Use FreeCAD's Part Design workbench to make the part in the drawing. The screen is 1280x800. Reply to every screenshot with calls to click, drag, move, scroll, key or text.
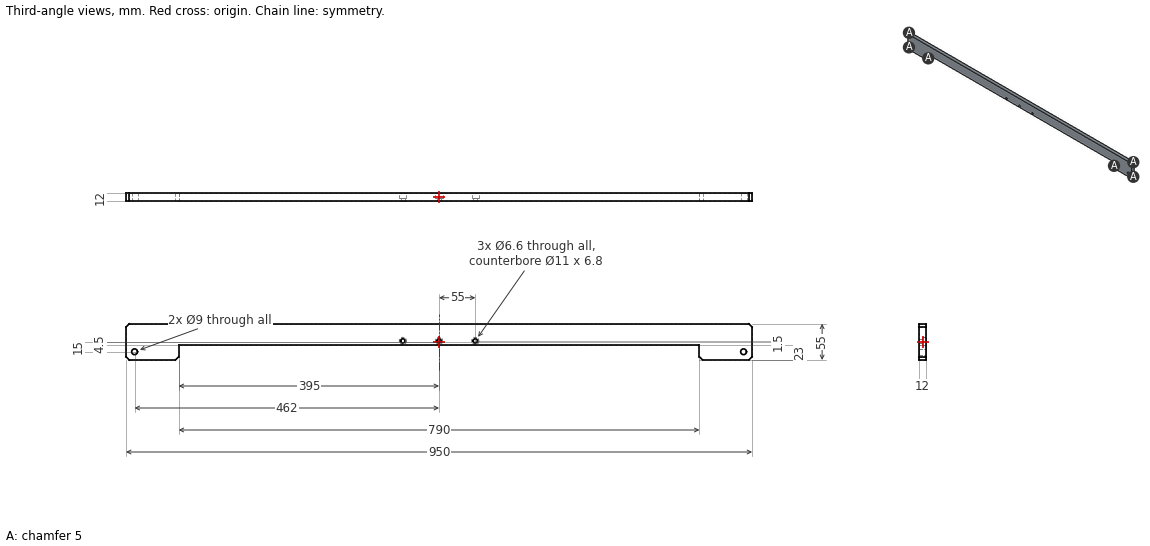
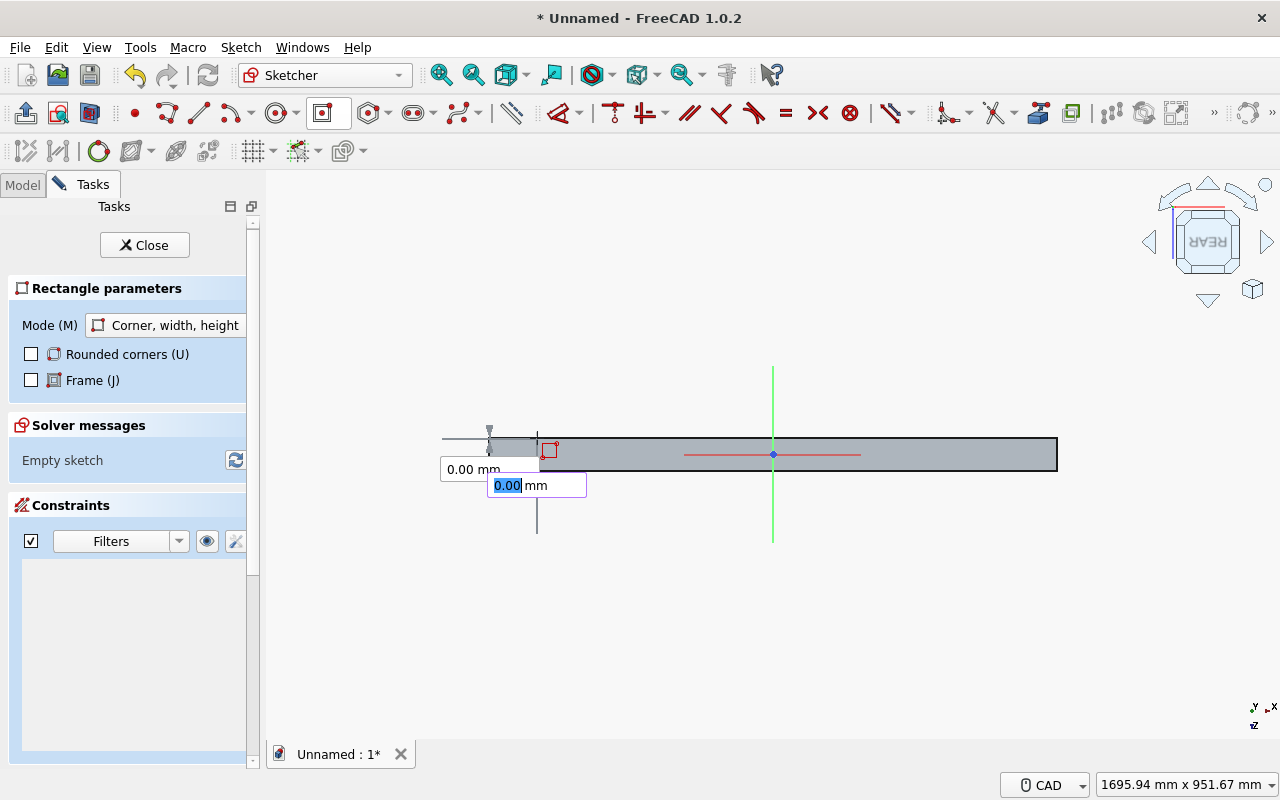
scroll(1009, 452, up, 9)
move(1006, 448)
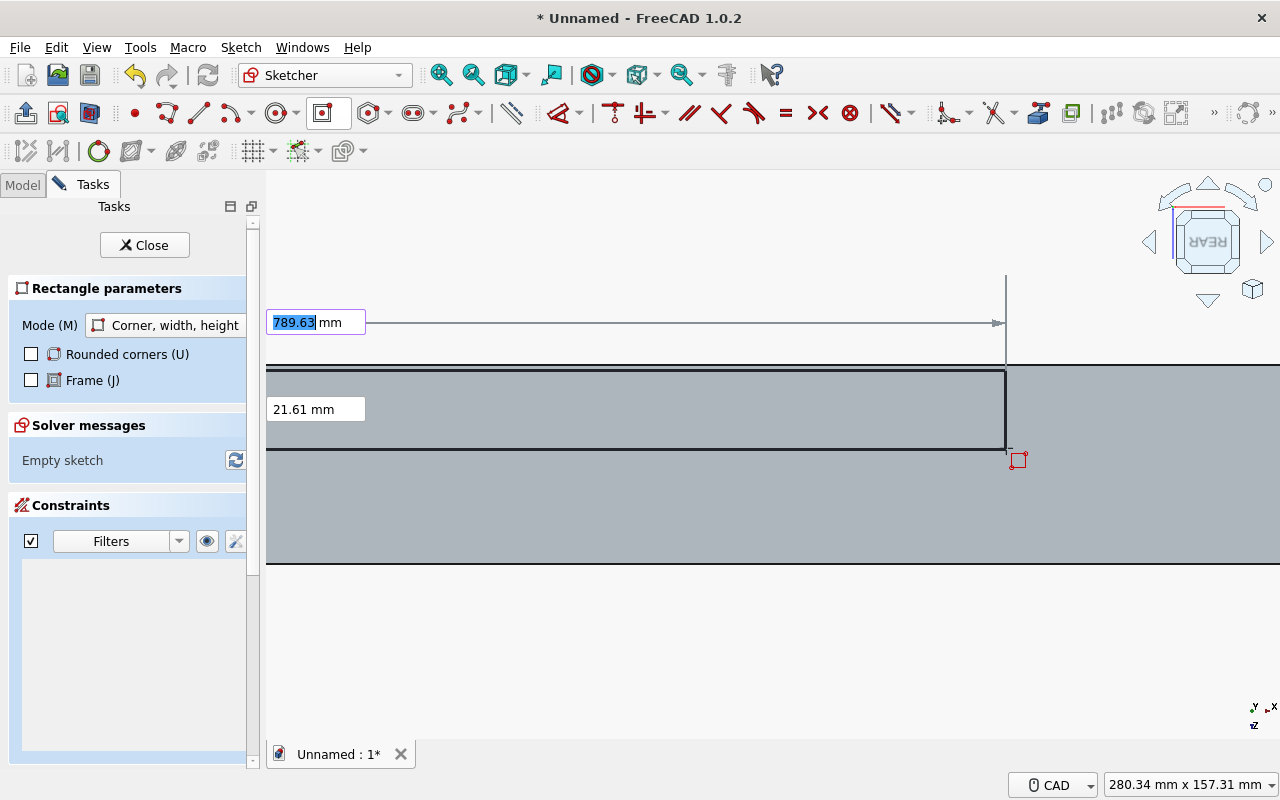
text(790)
key(Tab)
text(23)
key(Return)
key(Escape)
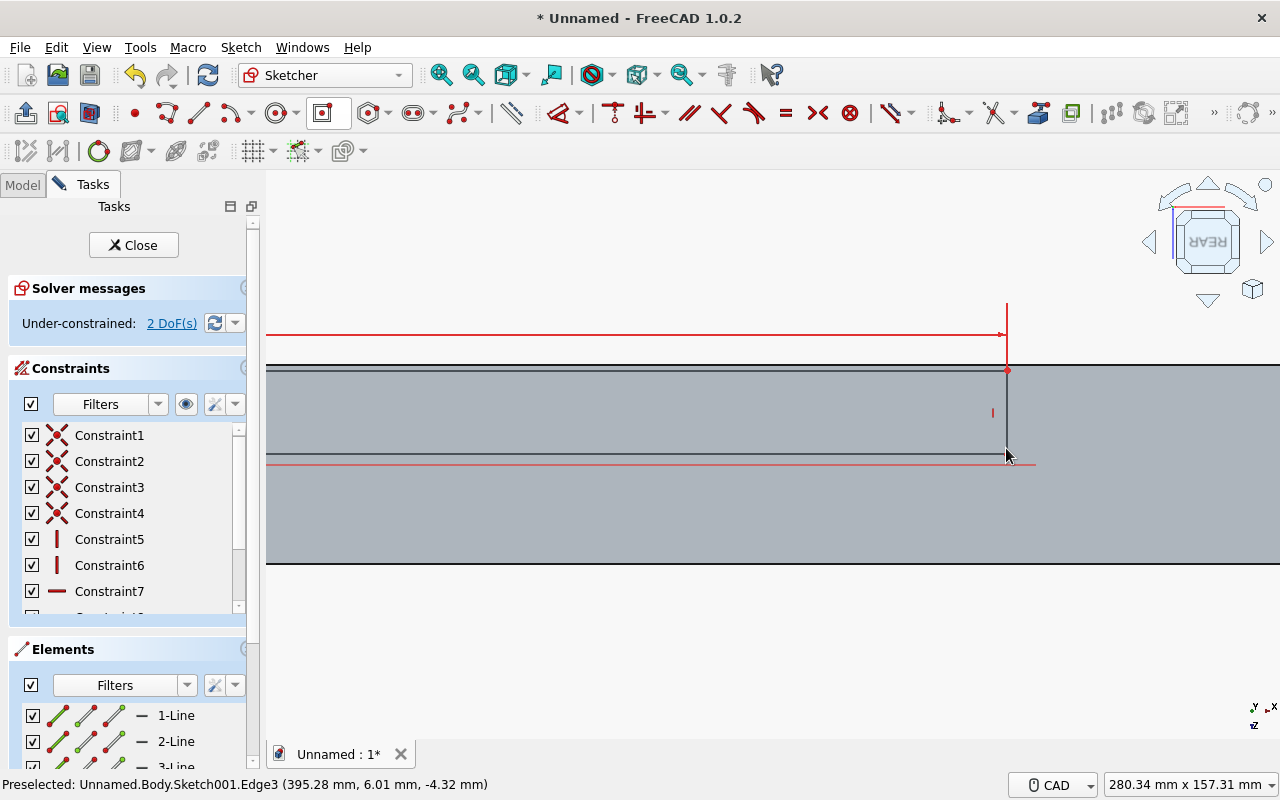
click(558, 114)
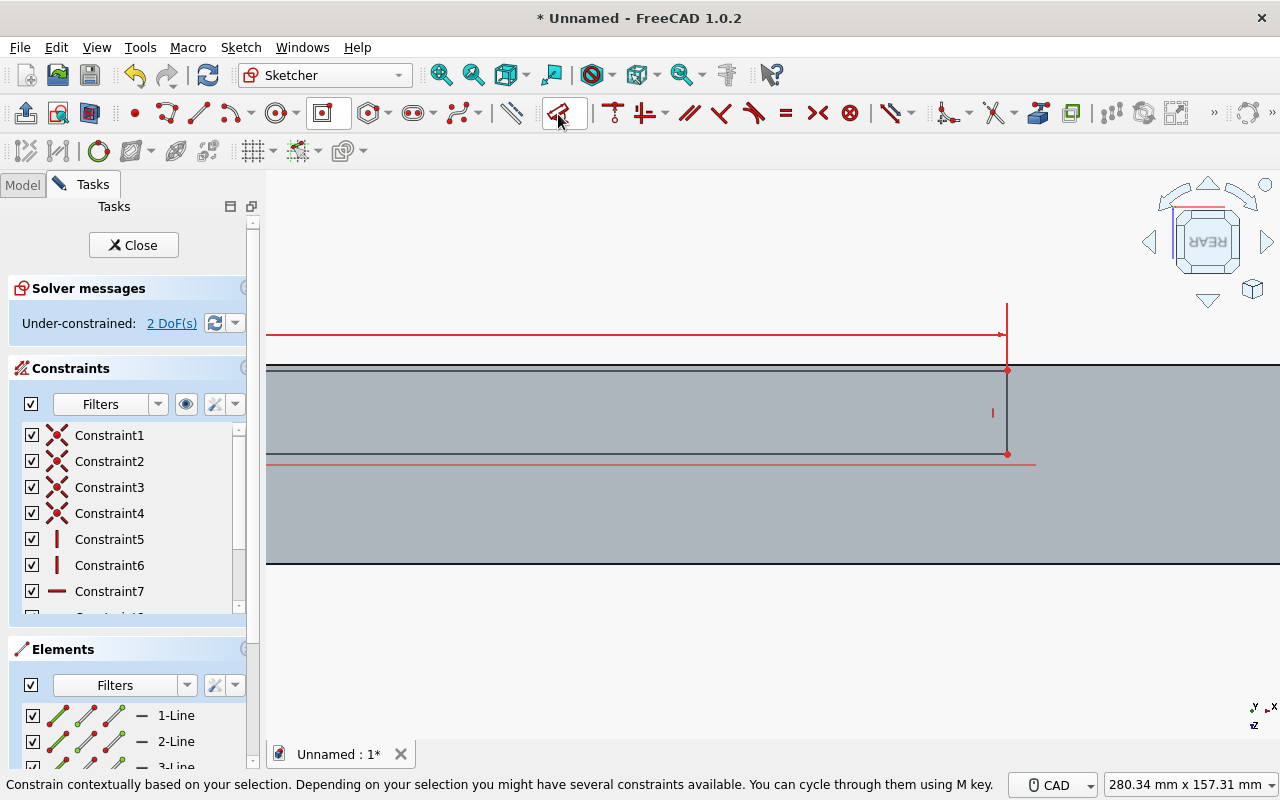
scroll(990, 465, down, 8)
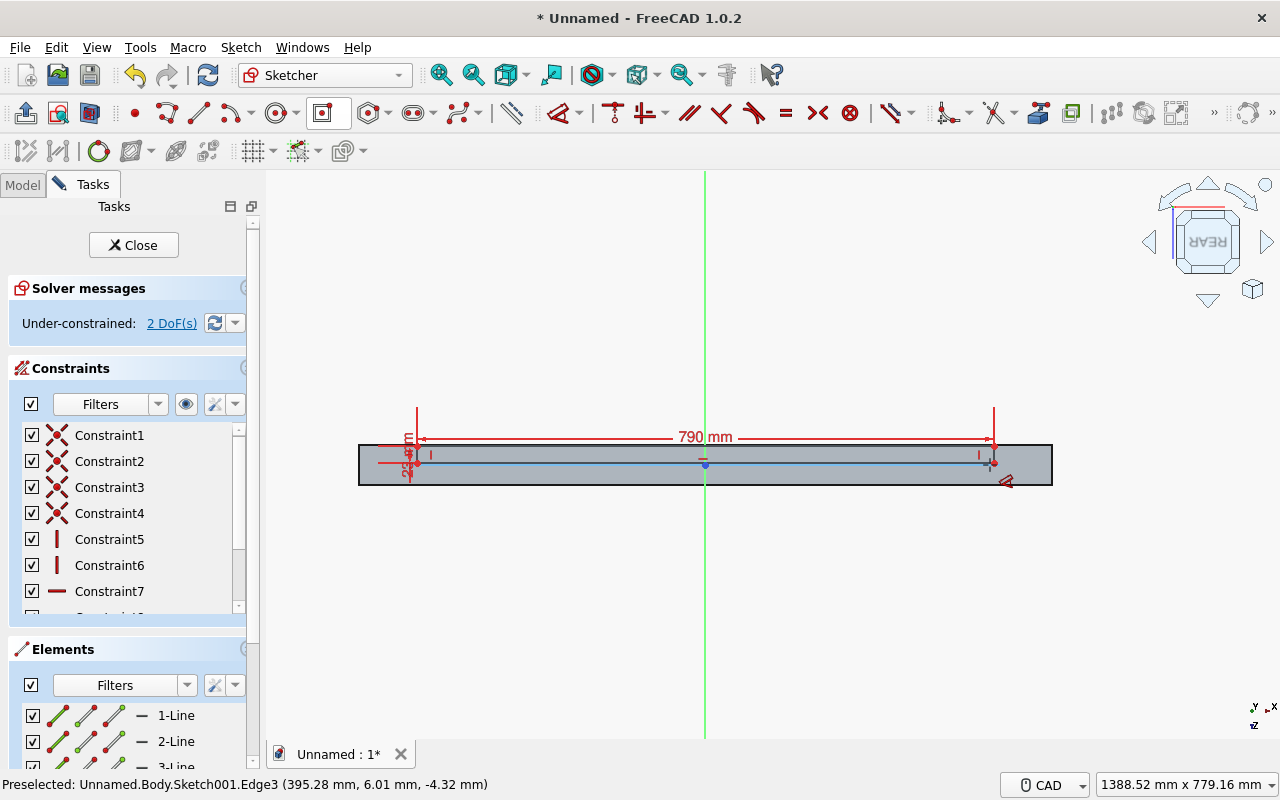
click(417, 446)
click(561, 499)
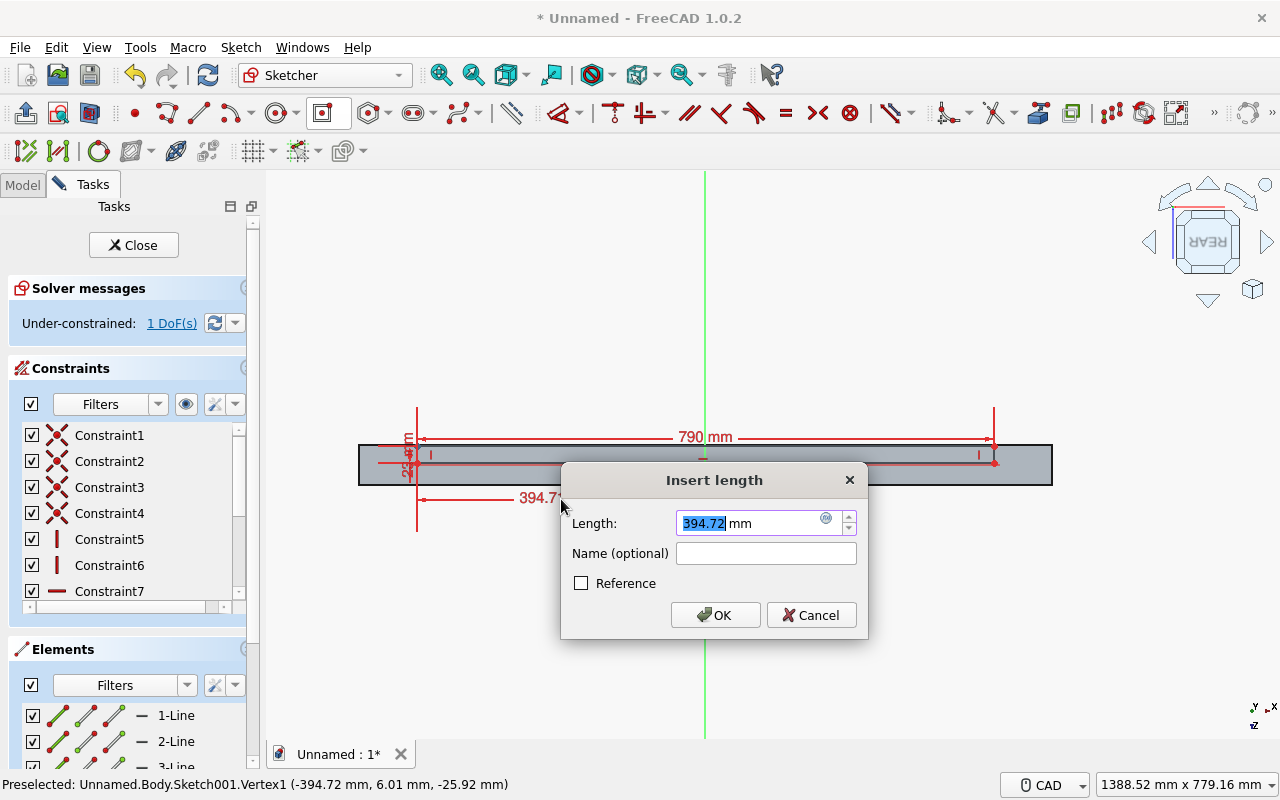
text(395)
key(Return)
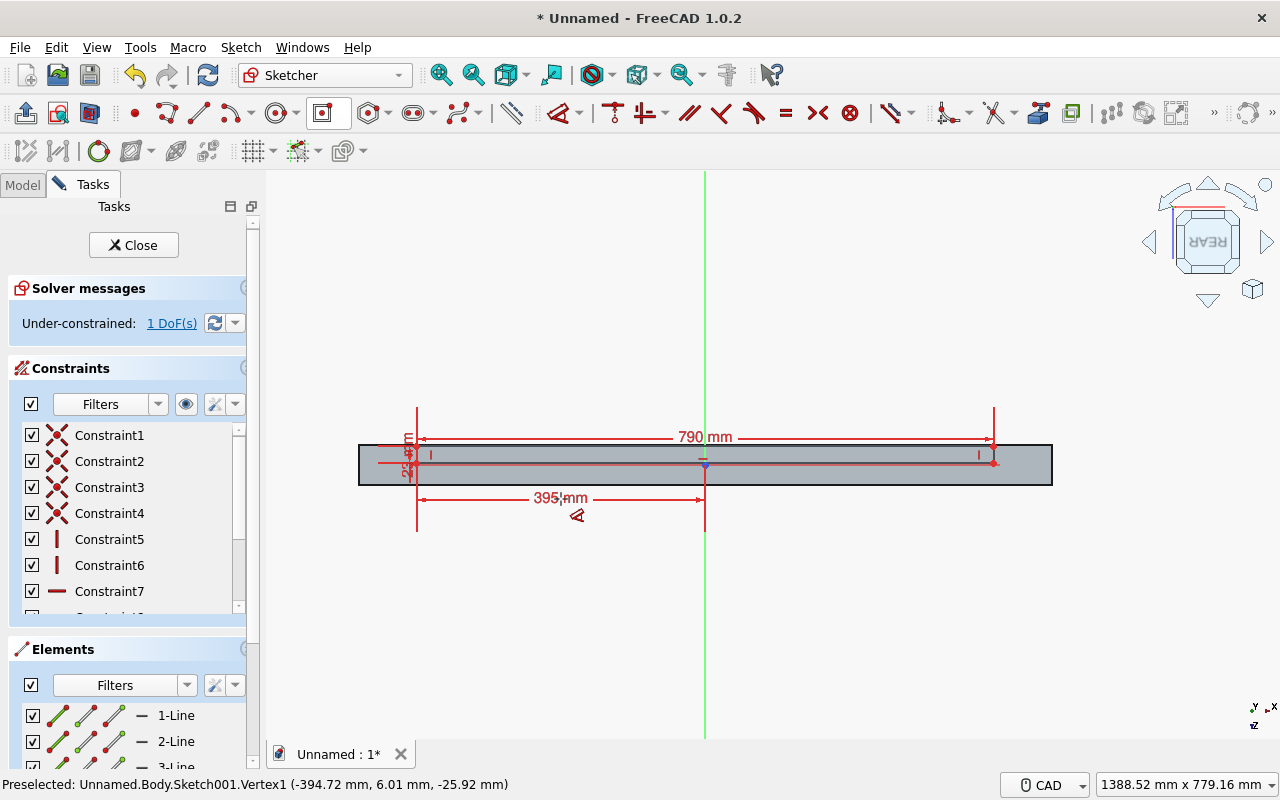
scroll(417, 463, up, 13)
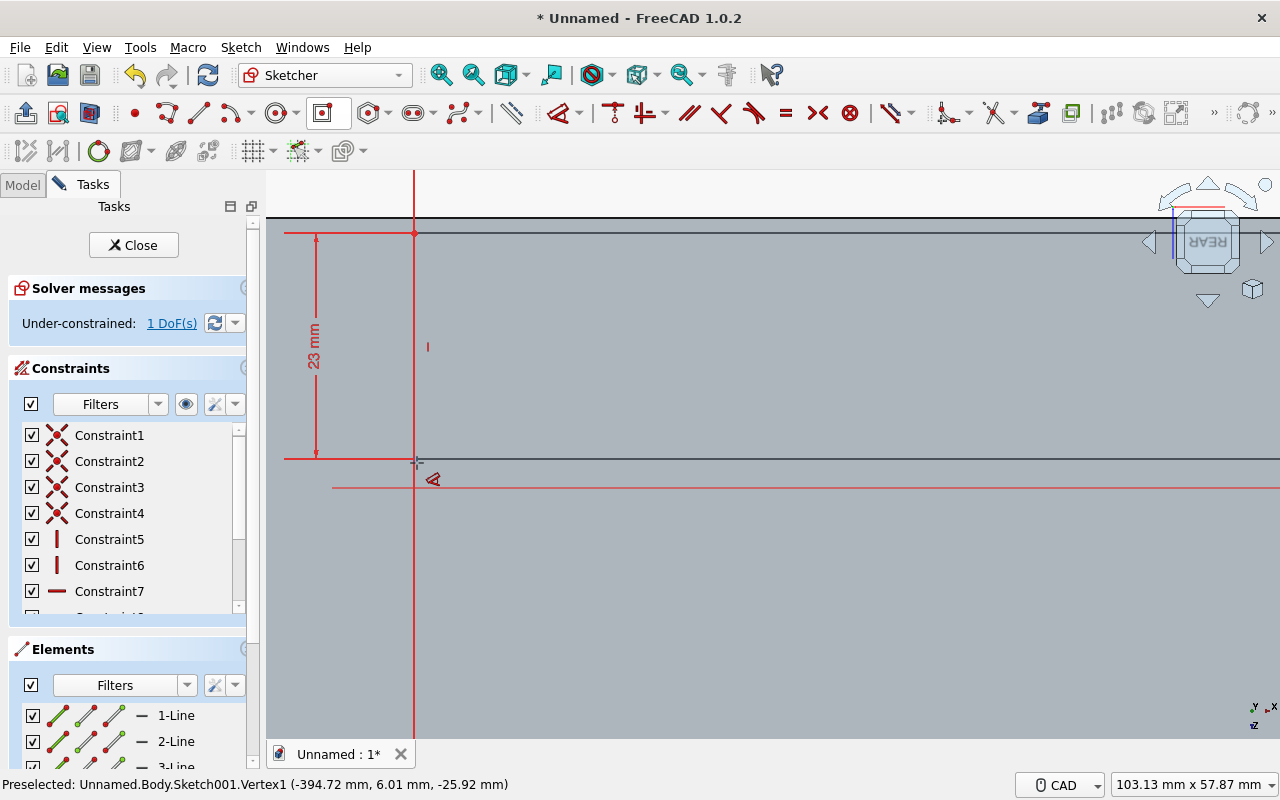
click(414, 459)
click(380, 474)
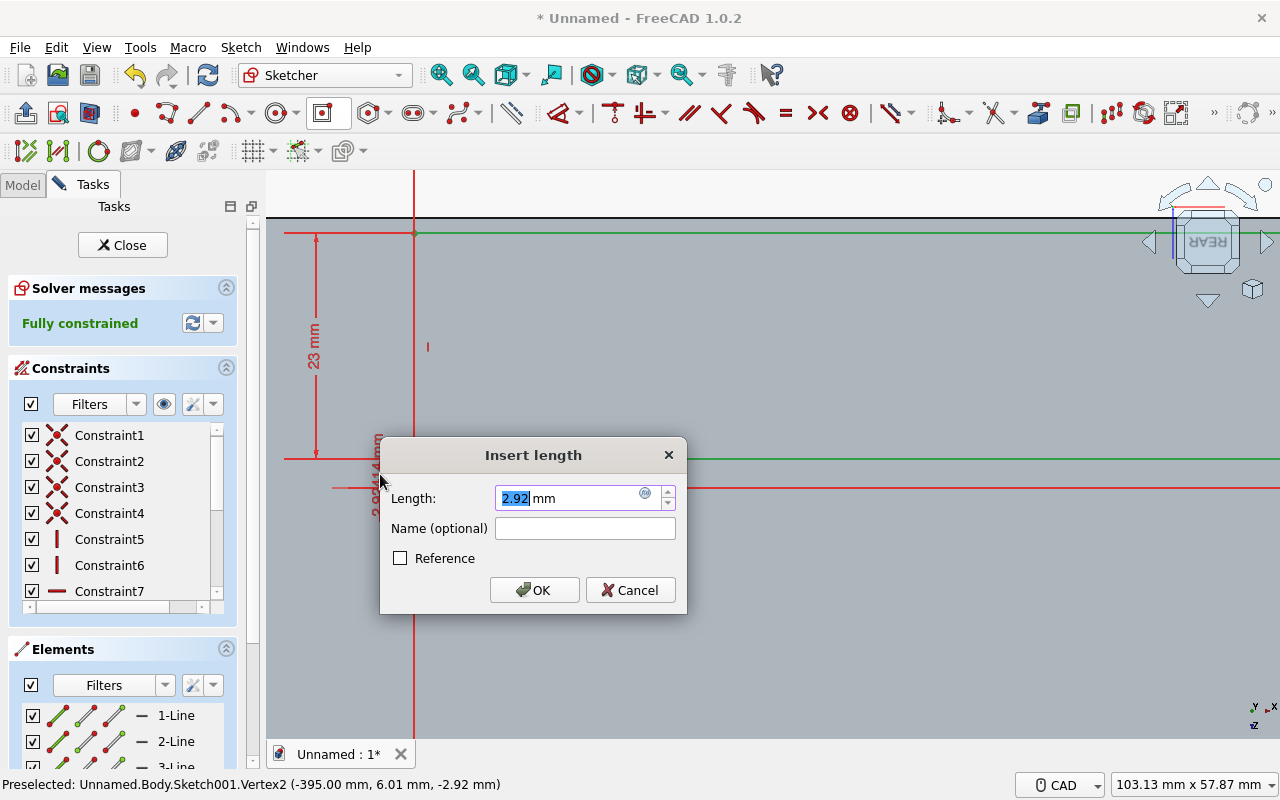
text(4.5)
key(Return)
key(Escape)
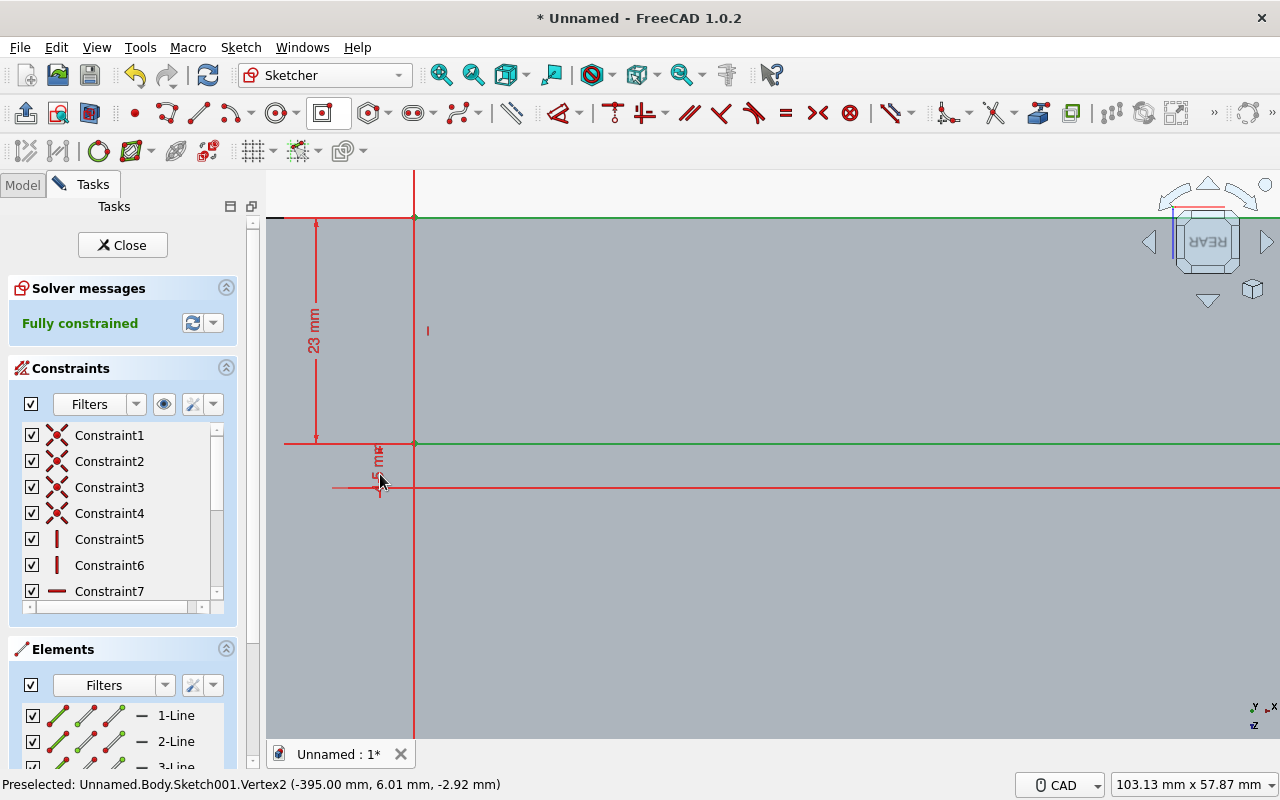
click(123, 245)